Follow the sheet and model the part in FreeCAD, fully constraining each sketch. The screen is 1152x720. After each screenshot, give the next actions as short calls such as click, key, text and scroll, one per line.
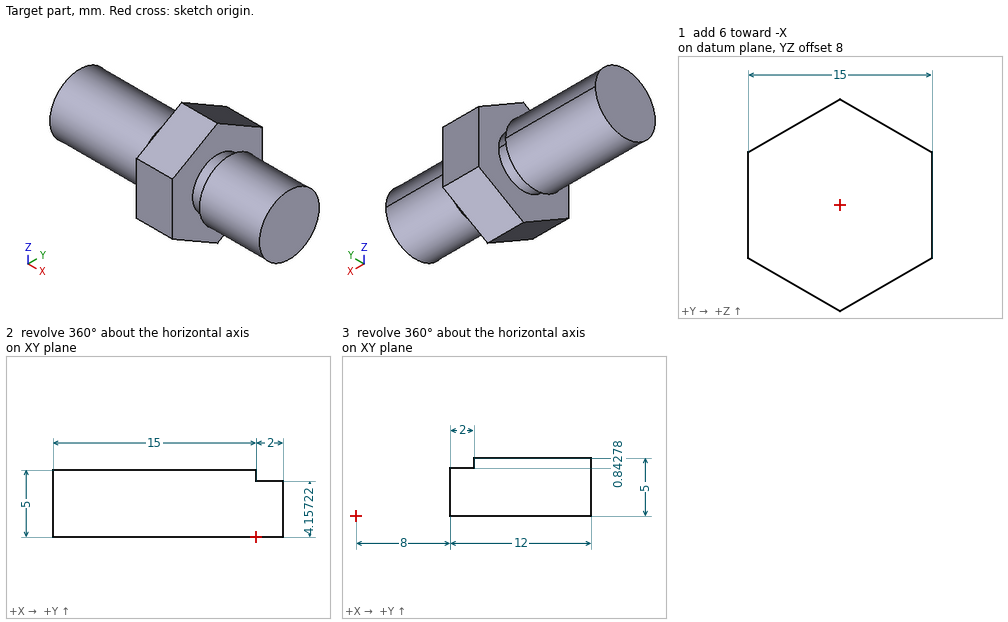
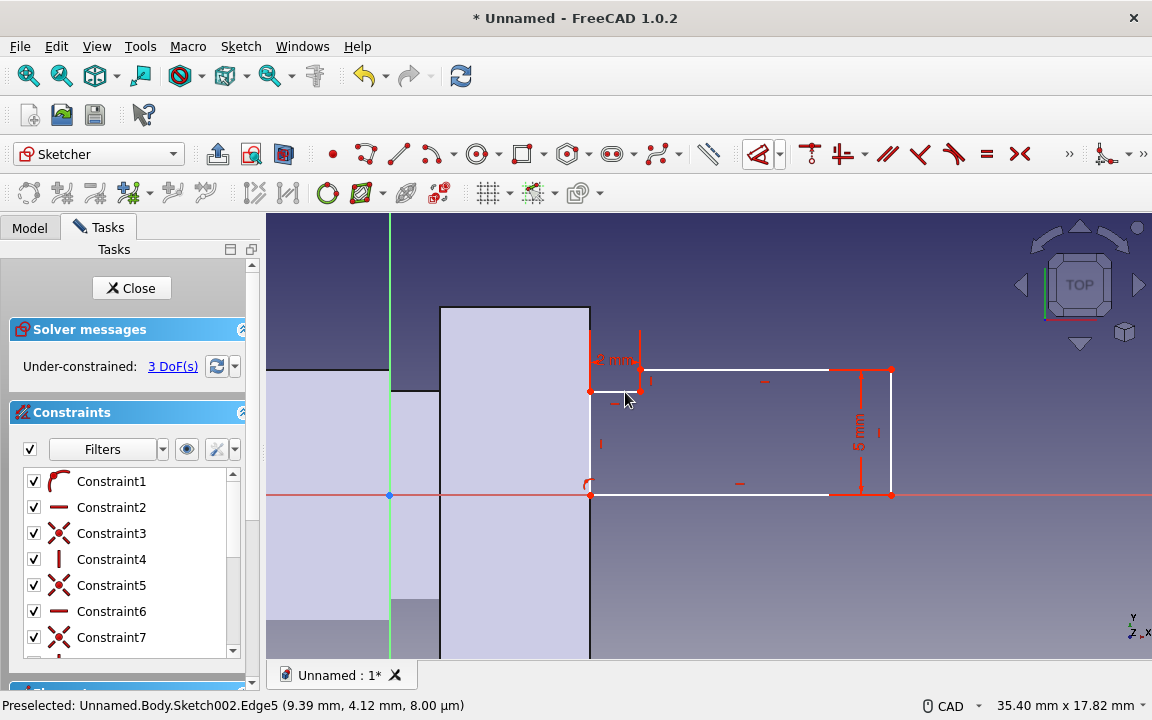
click(680, 495)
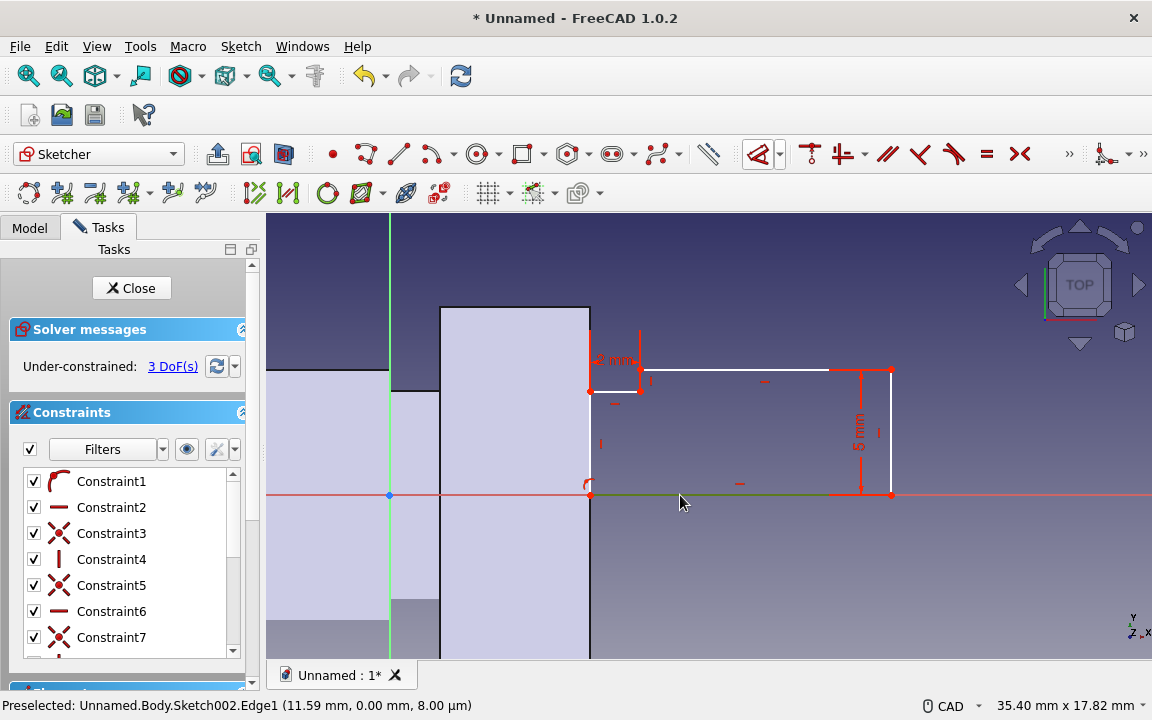
key(l)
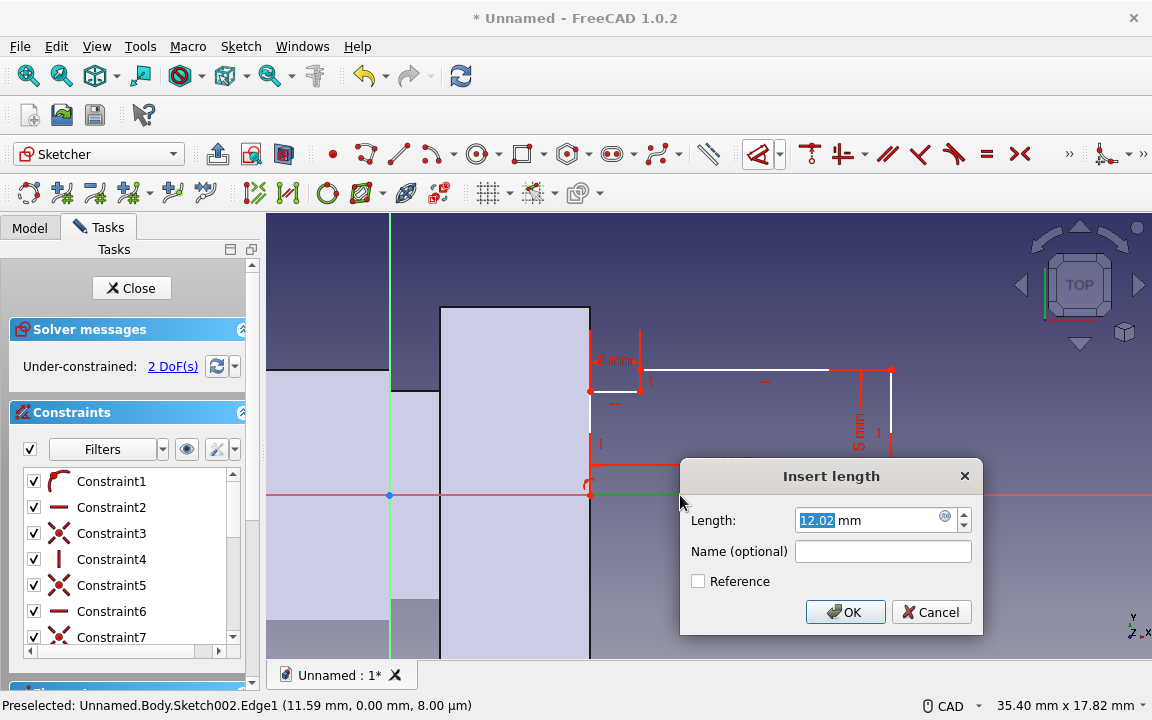
text(12)
key(Return)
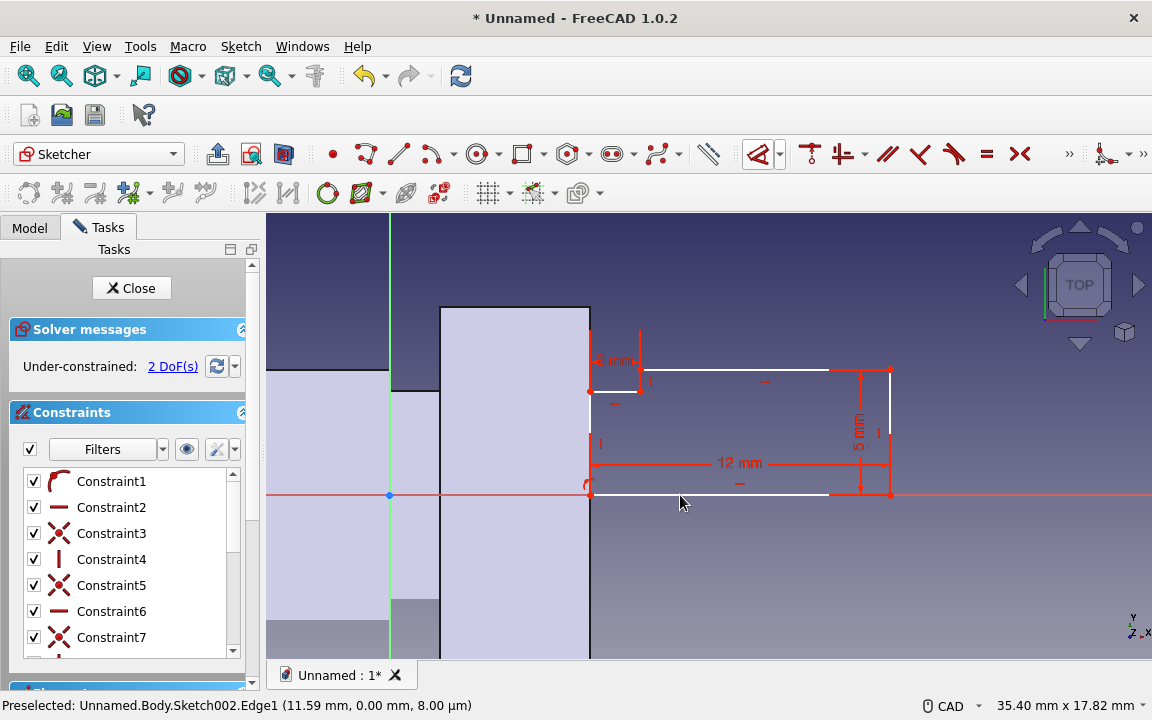
click(590, 495)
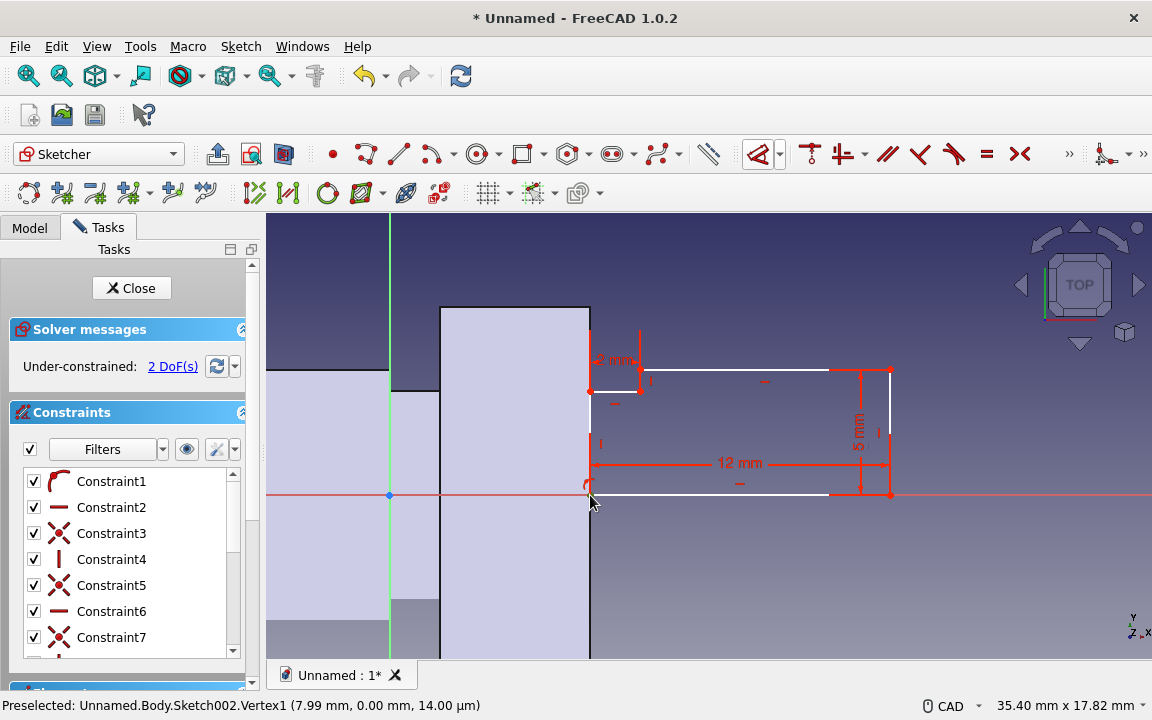
click(780, 154)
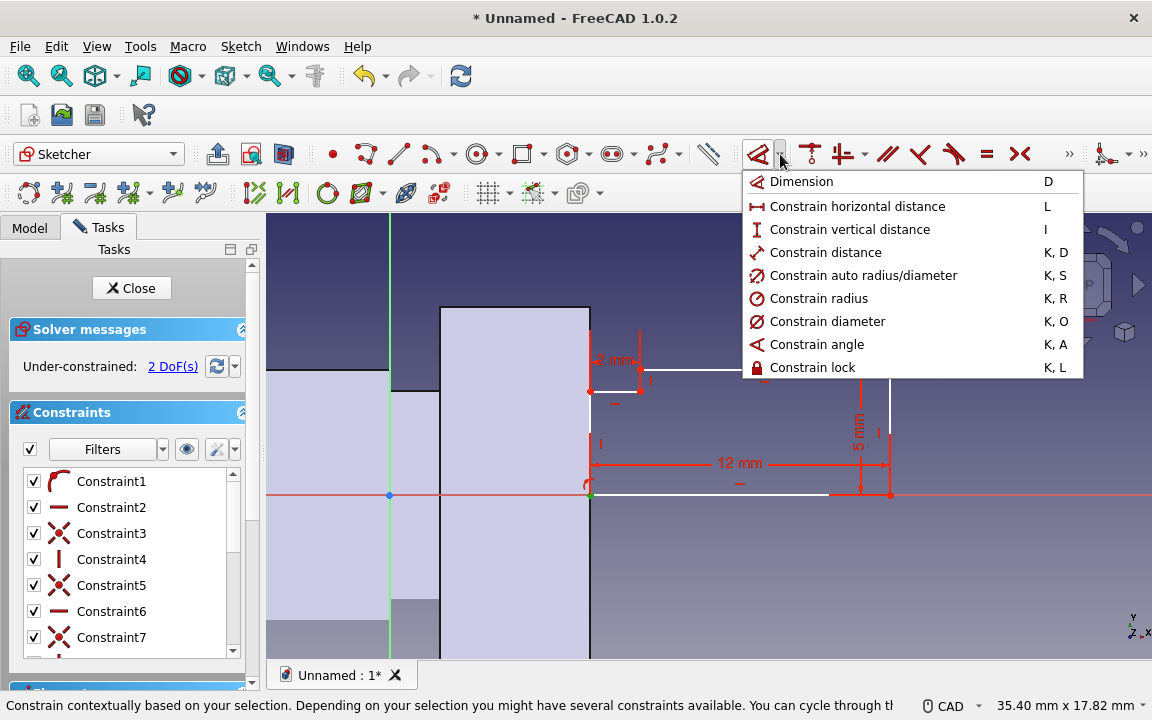
click(913, 206)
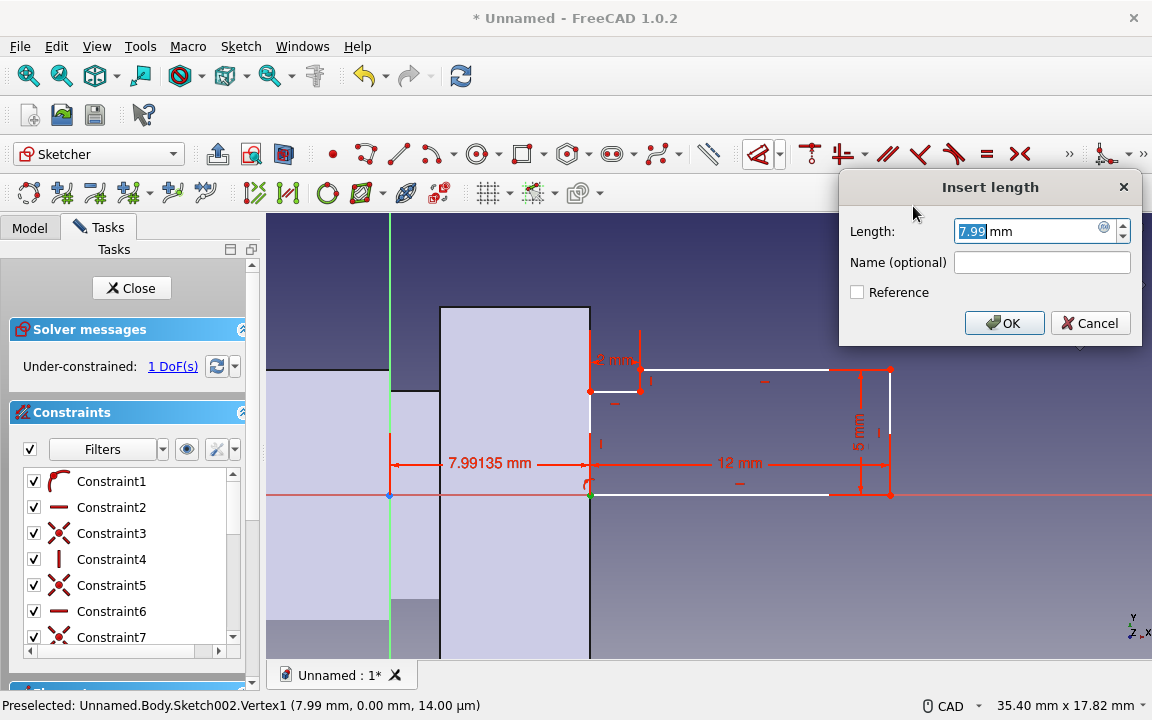
text(8)
key(Return)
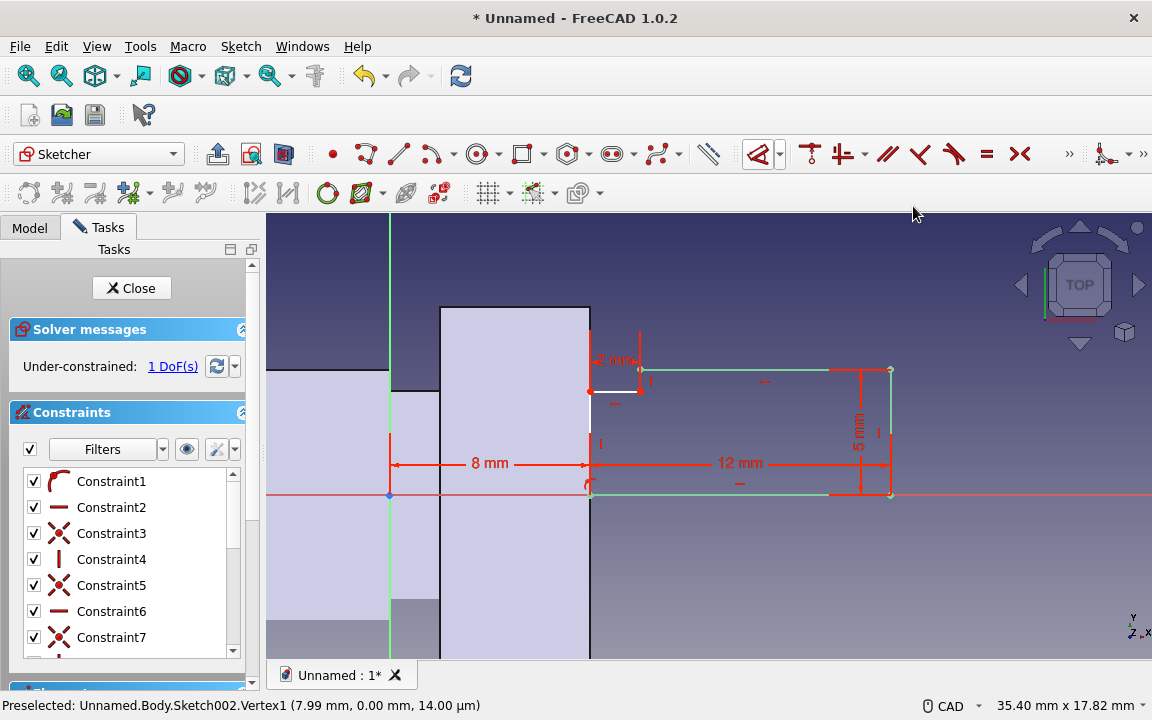
scroll(640, 381, up, 4)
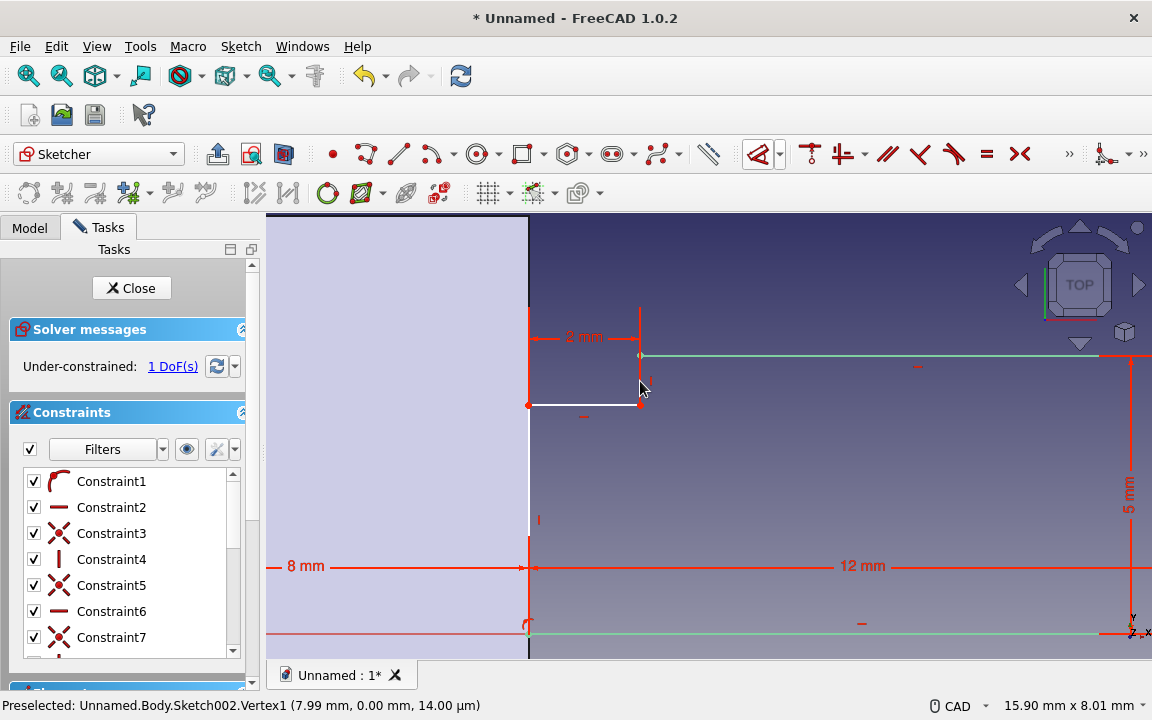
click(640, 380)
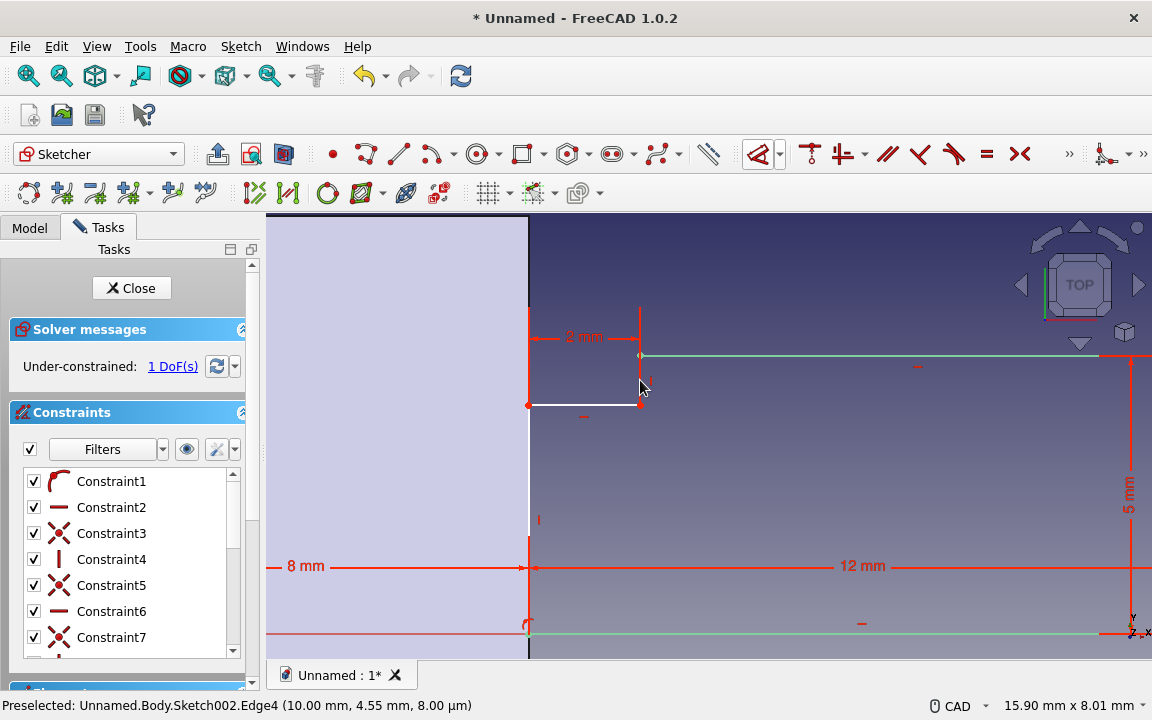
key(i)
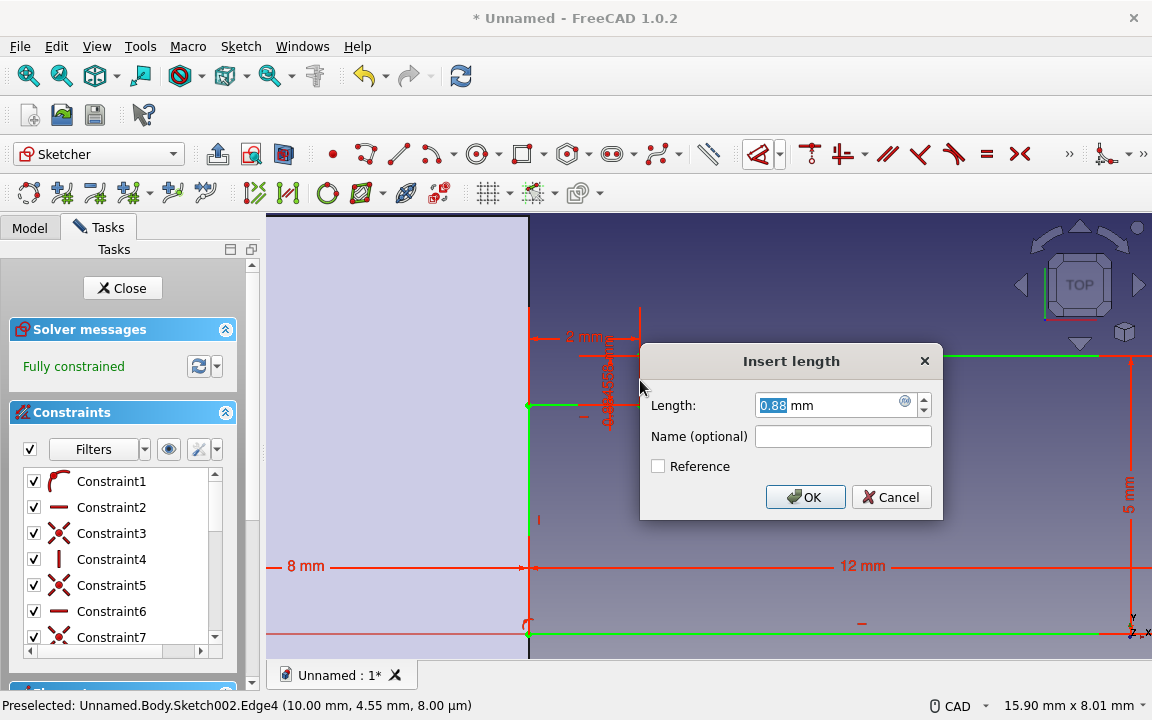
text(0.84278)
key(Return)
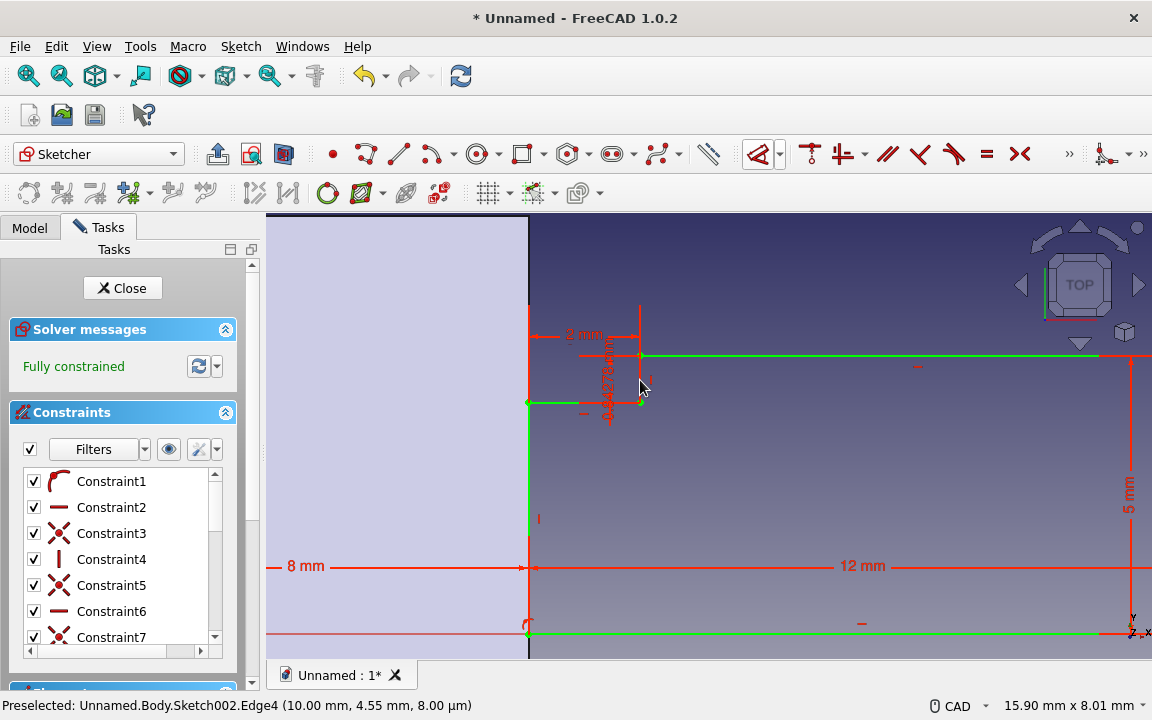
click(123, 288)